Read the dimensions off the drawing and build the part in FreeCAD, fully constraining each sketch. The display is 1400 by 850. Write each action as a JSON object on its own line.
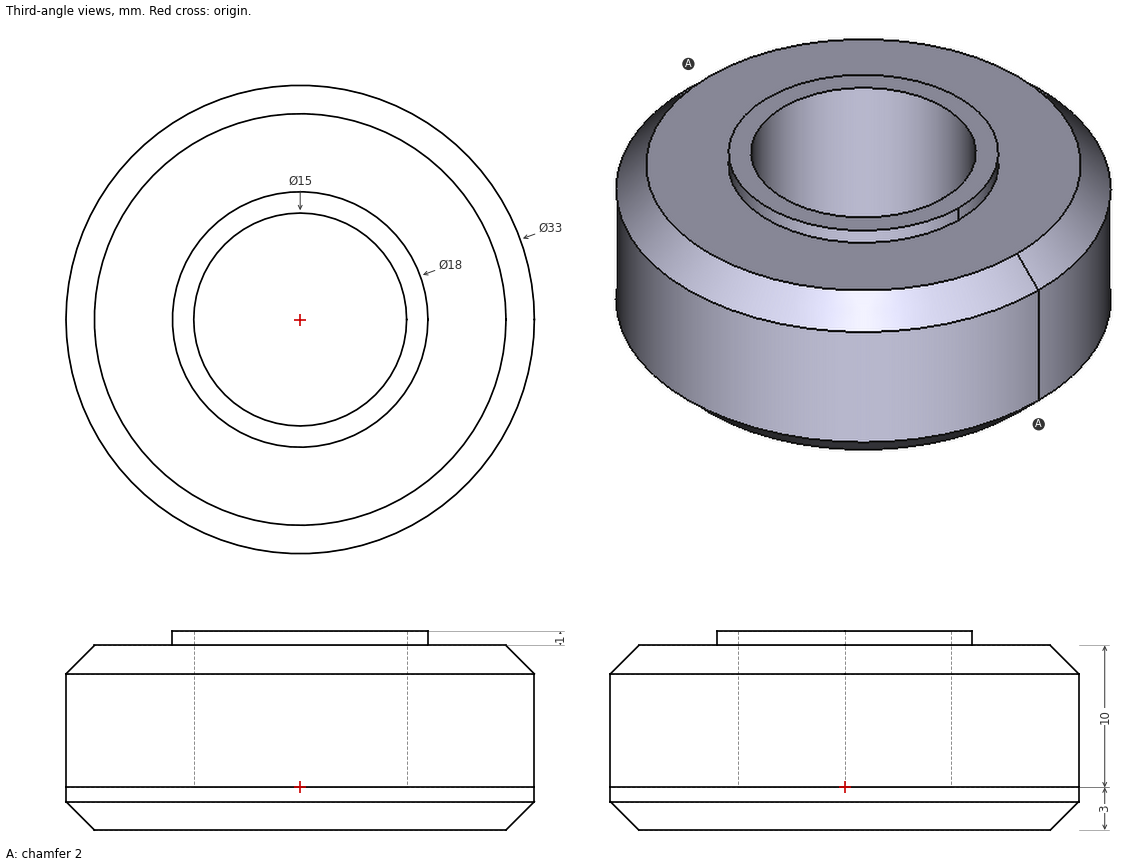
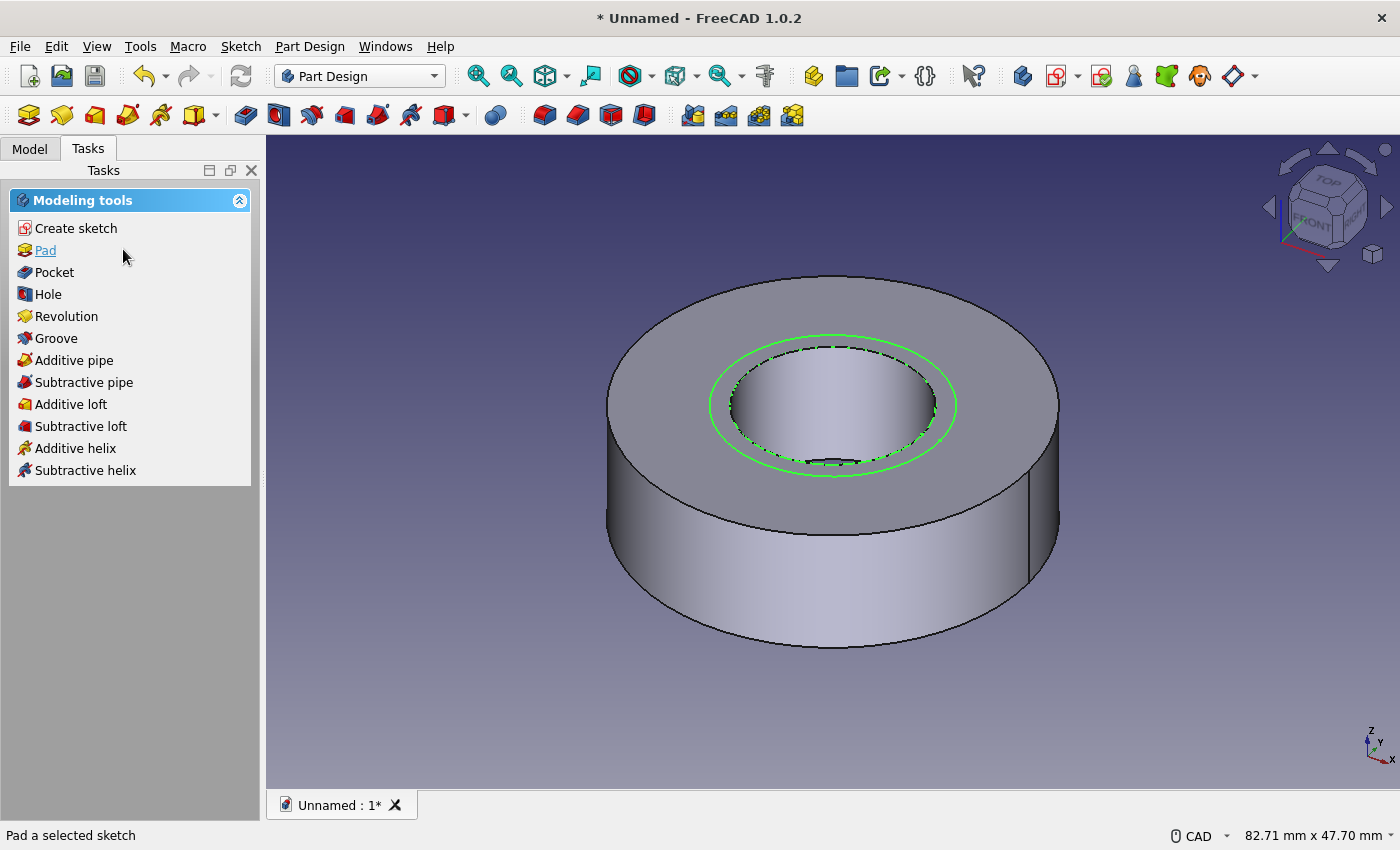
{"action": "left_click", "coordinate": [29, 116]}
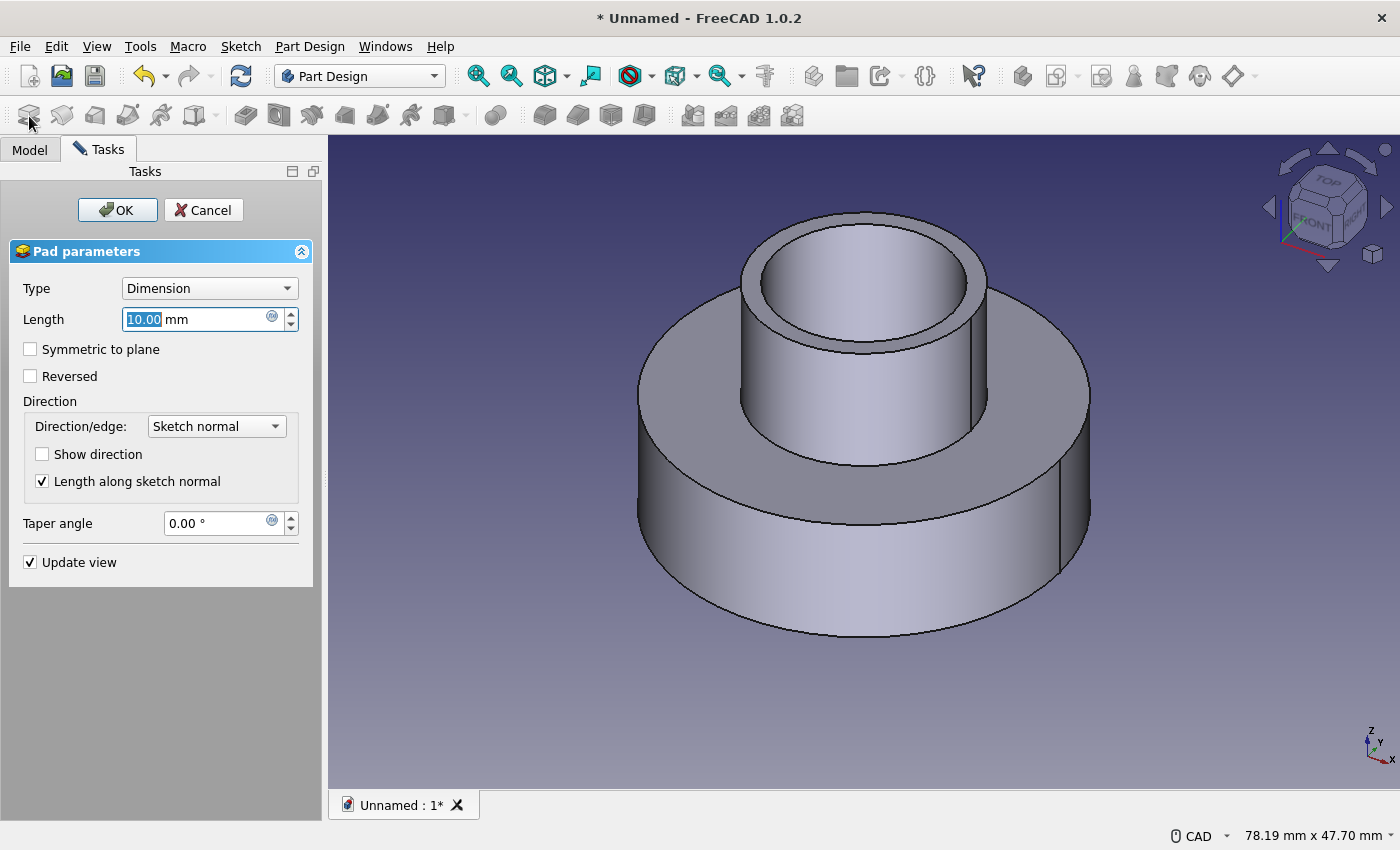
{"action": "type", "text": "1"}
{"action": "key", "text": "Tab"}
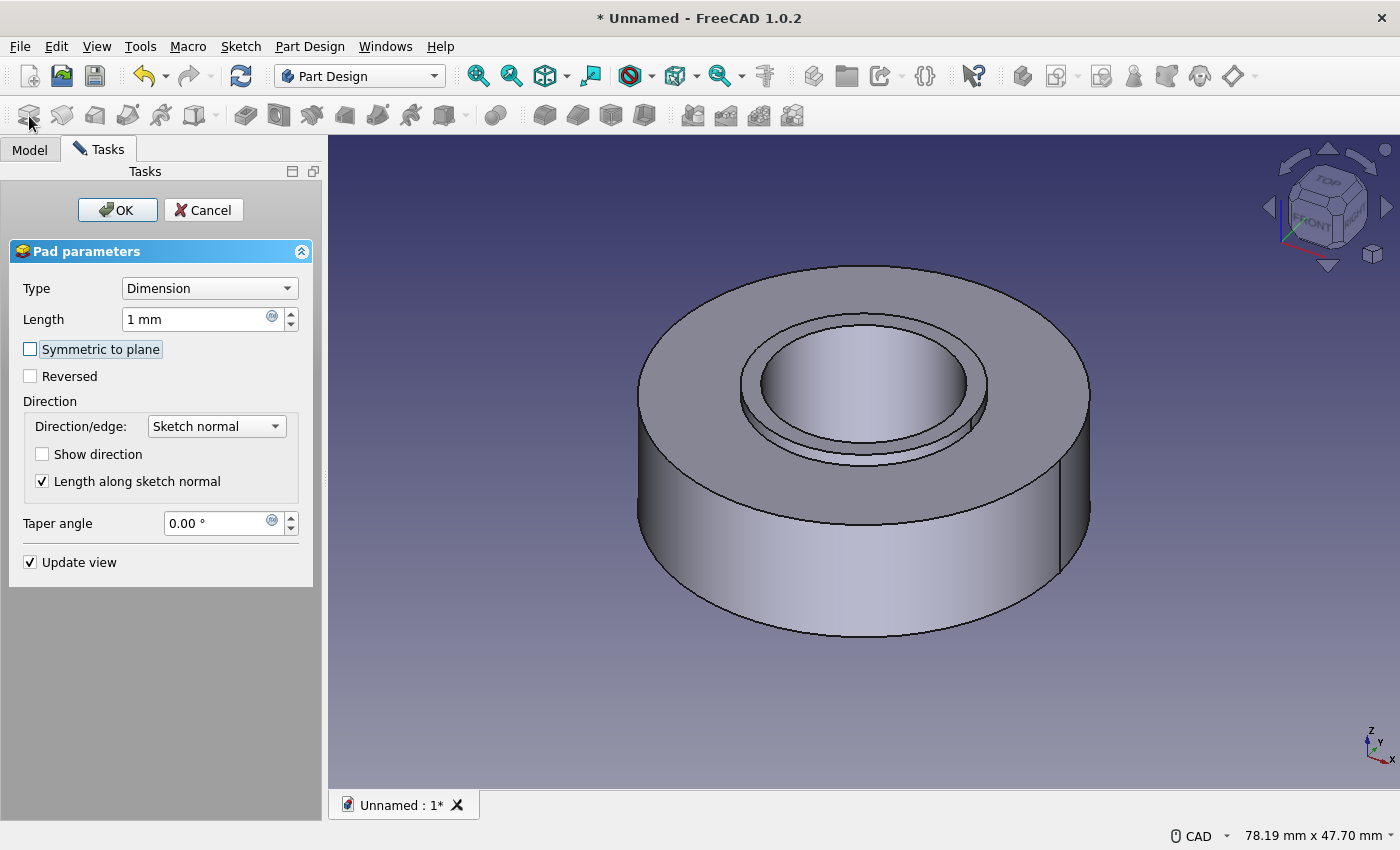
{"action": "left_click", "coordinate": [118, 210]}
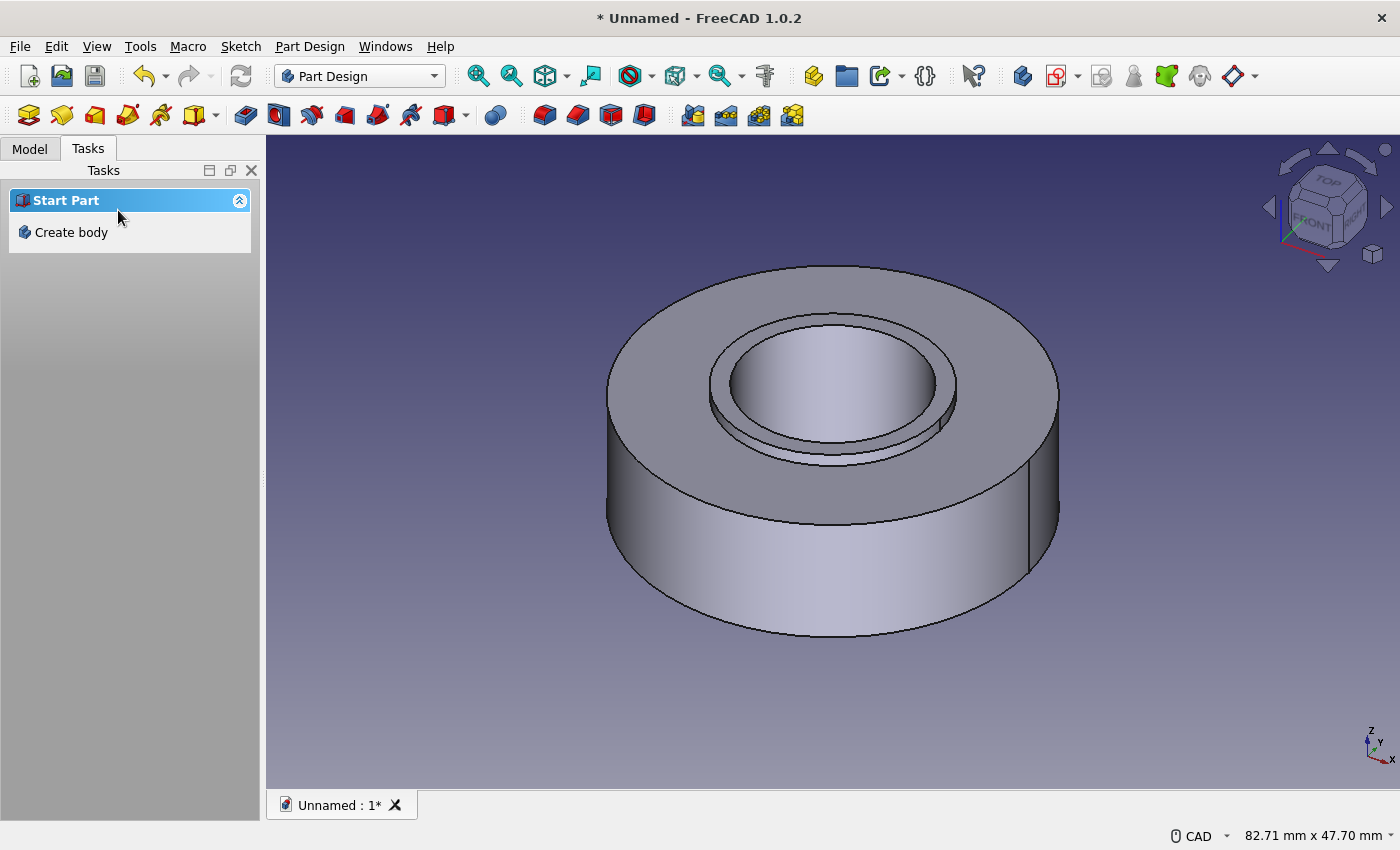
{"action": "left_click", "coordinate": [30, 148]}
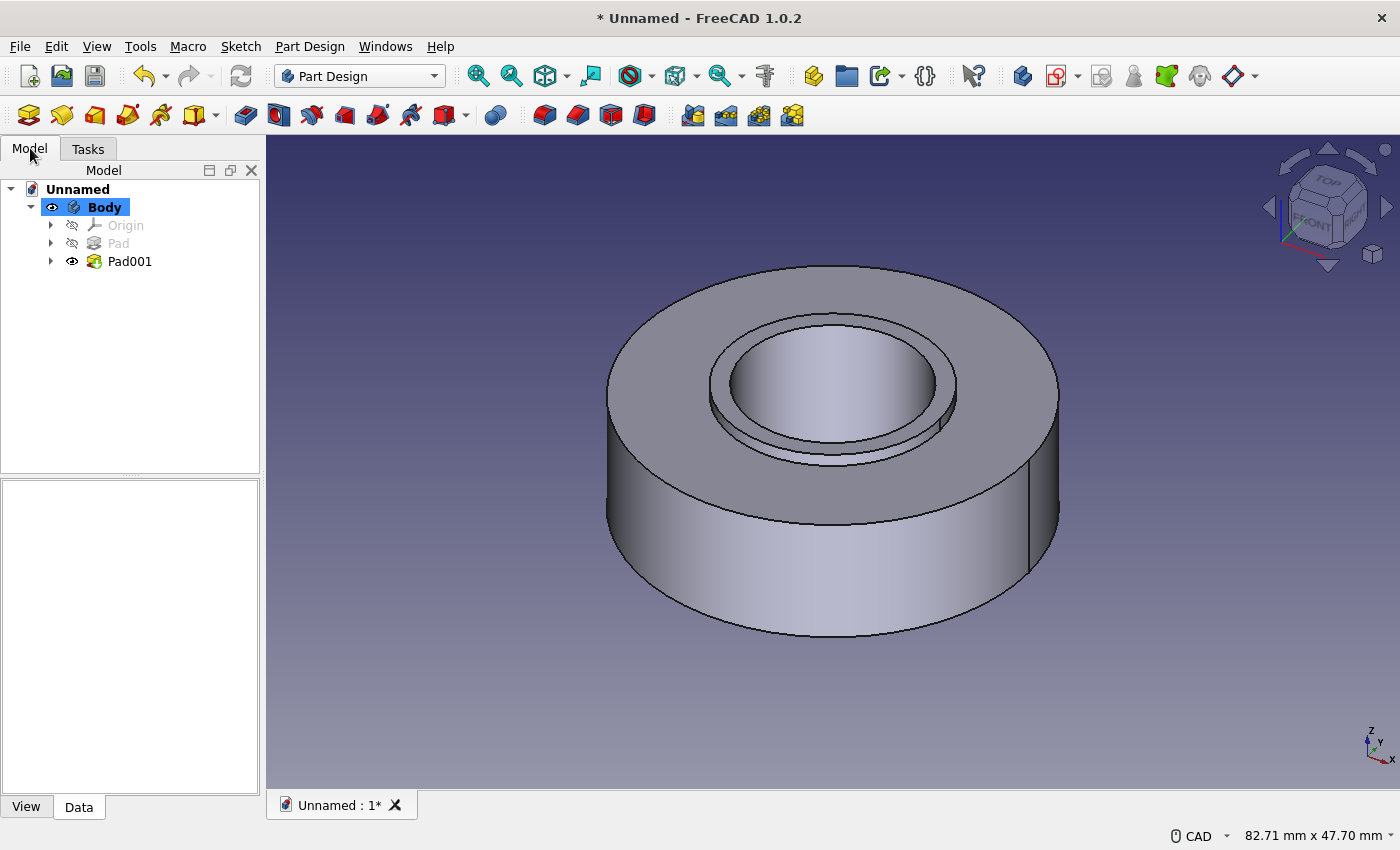
{"action": "left_click", "coordinate": [51, 225]}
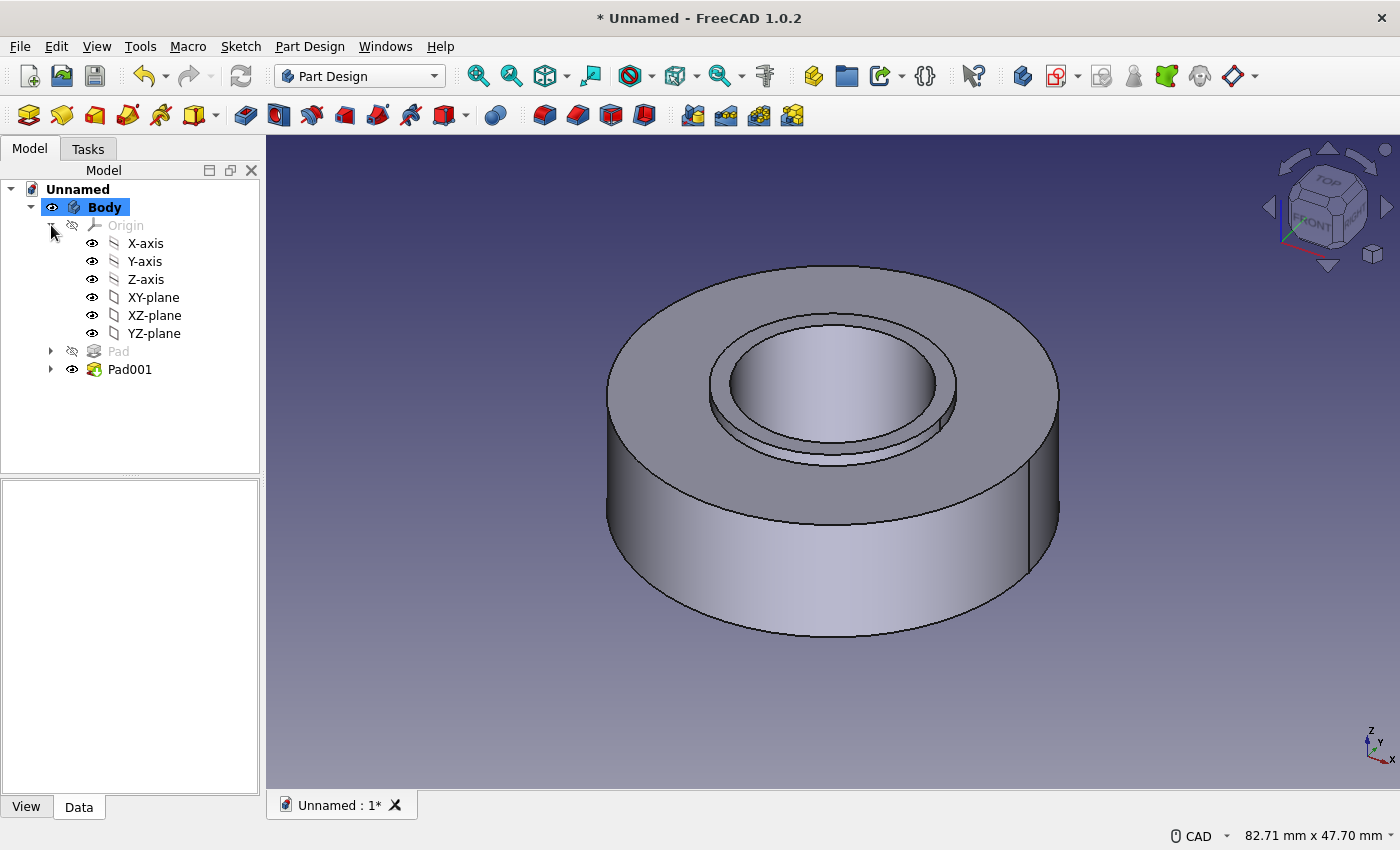
{"action": "left_click", "coordinate": [137, 297]}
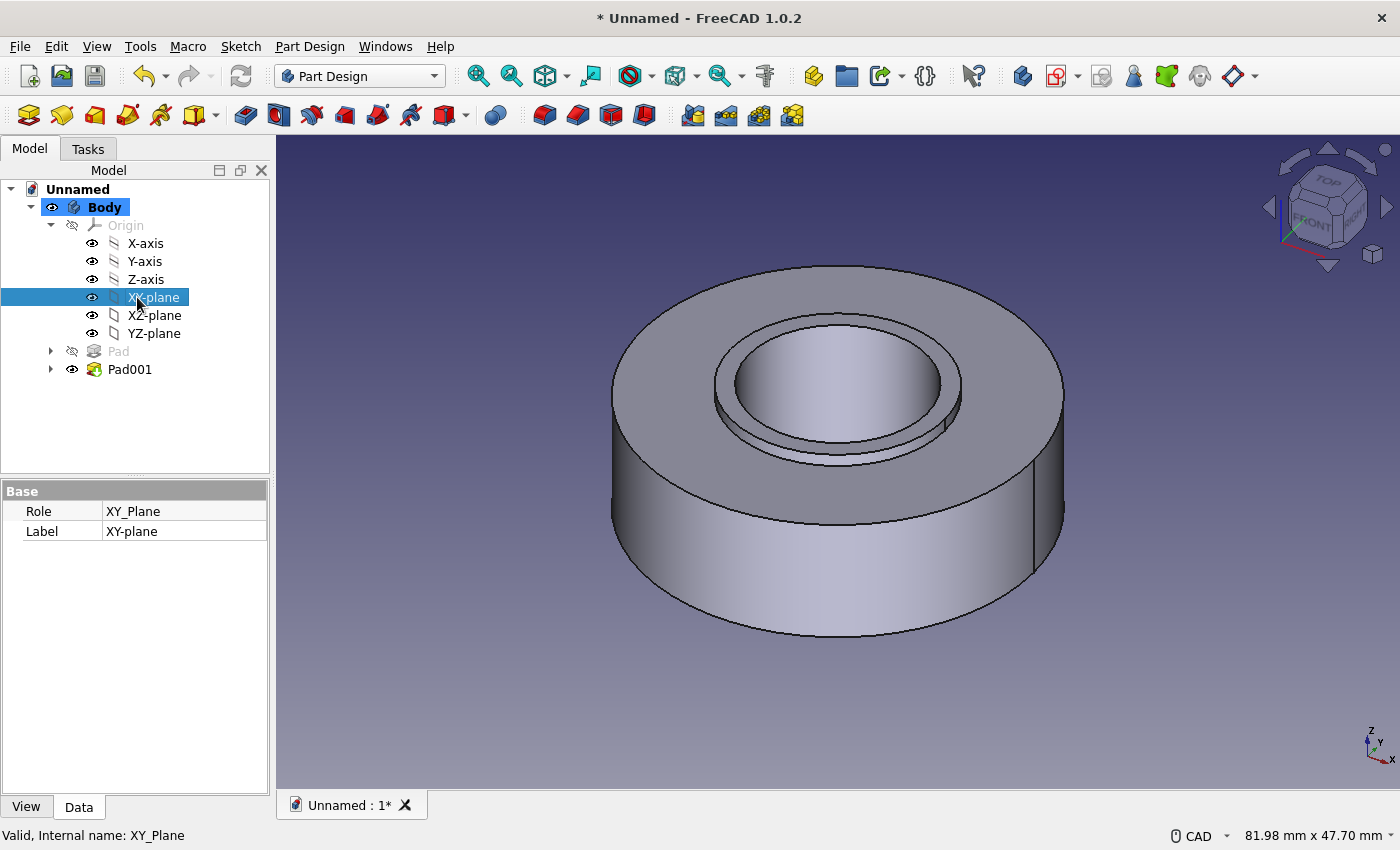
{"action": "left_click", "coordinate": [1232, 76]}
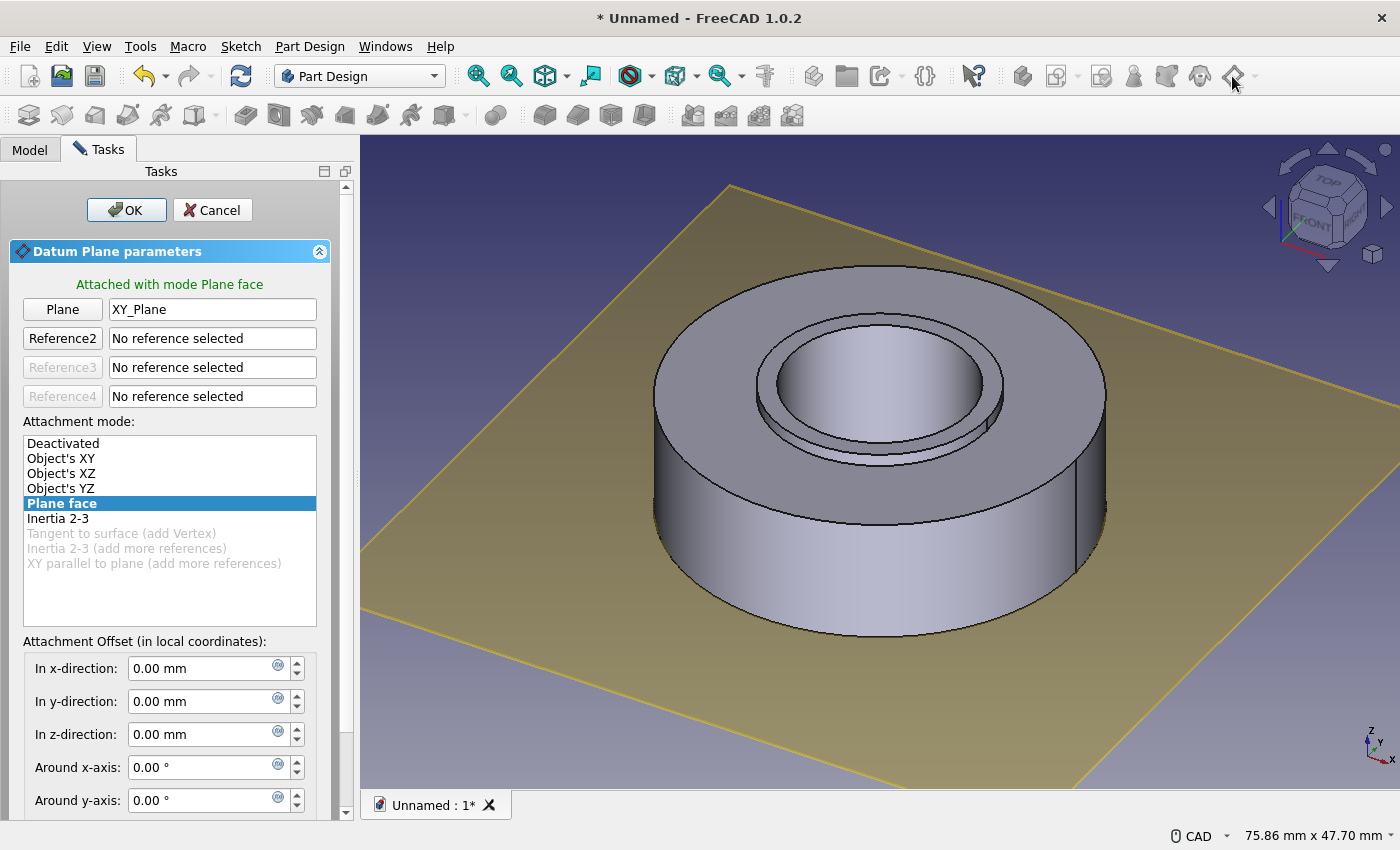
{"action": "triple_click", "coordinate": [210, 734]}